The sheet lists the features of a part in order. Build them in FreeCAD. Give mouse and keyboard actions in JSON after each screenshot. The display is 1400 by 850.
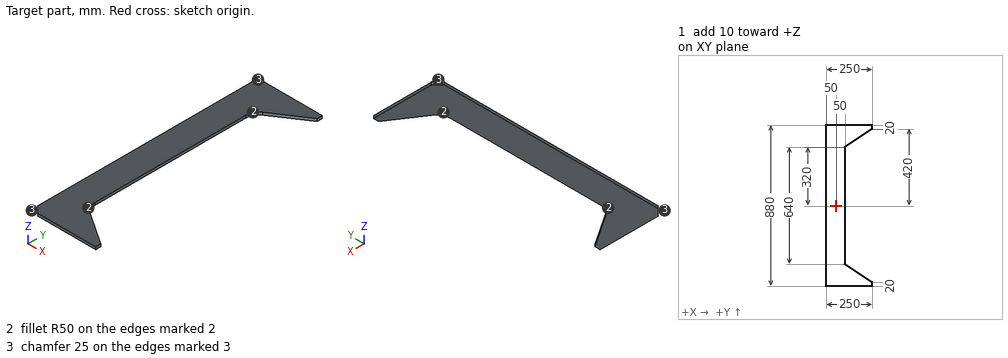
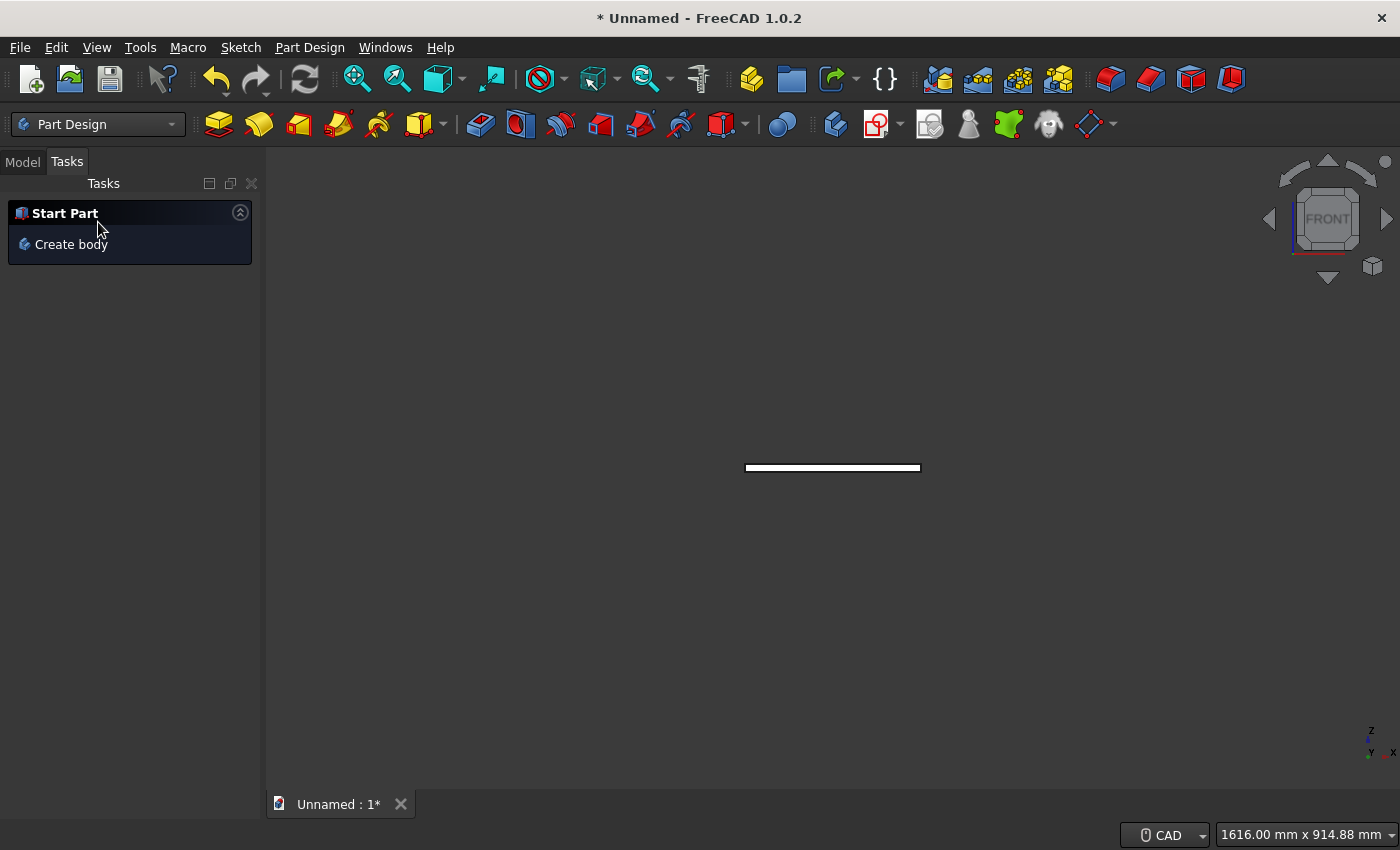
{"action": "scroll", "coordinate": [745, 467], "scroll_direction": "up", "scroll_amount": 9}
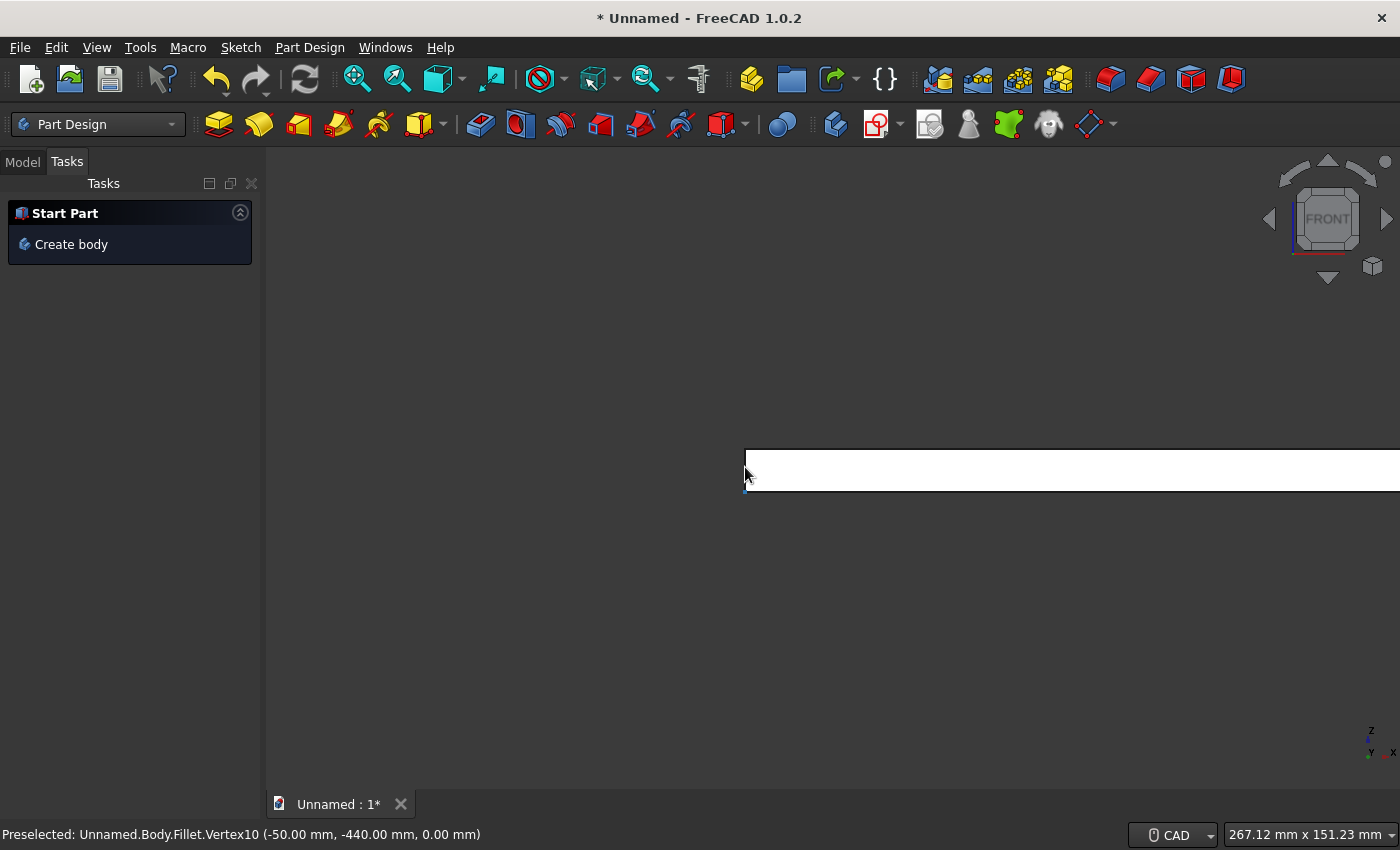
{"action": "left_click", "coordinate": [745, 470]}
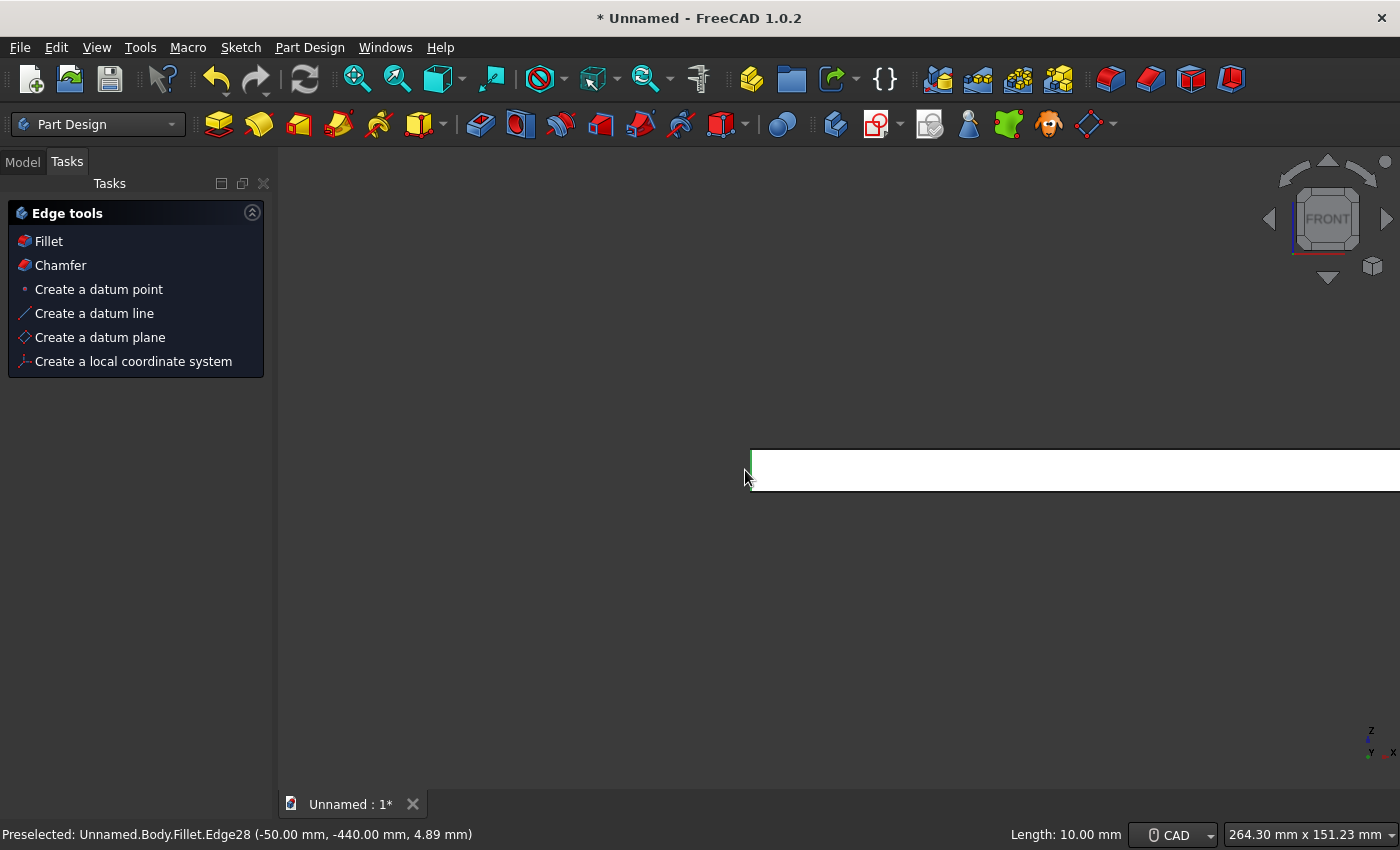
{"action": "left_click", "coordinate": [358, 80]}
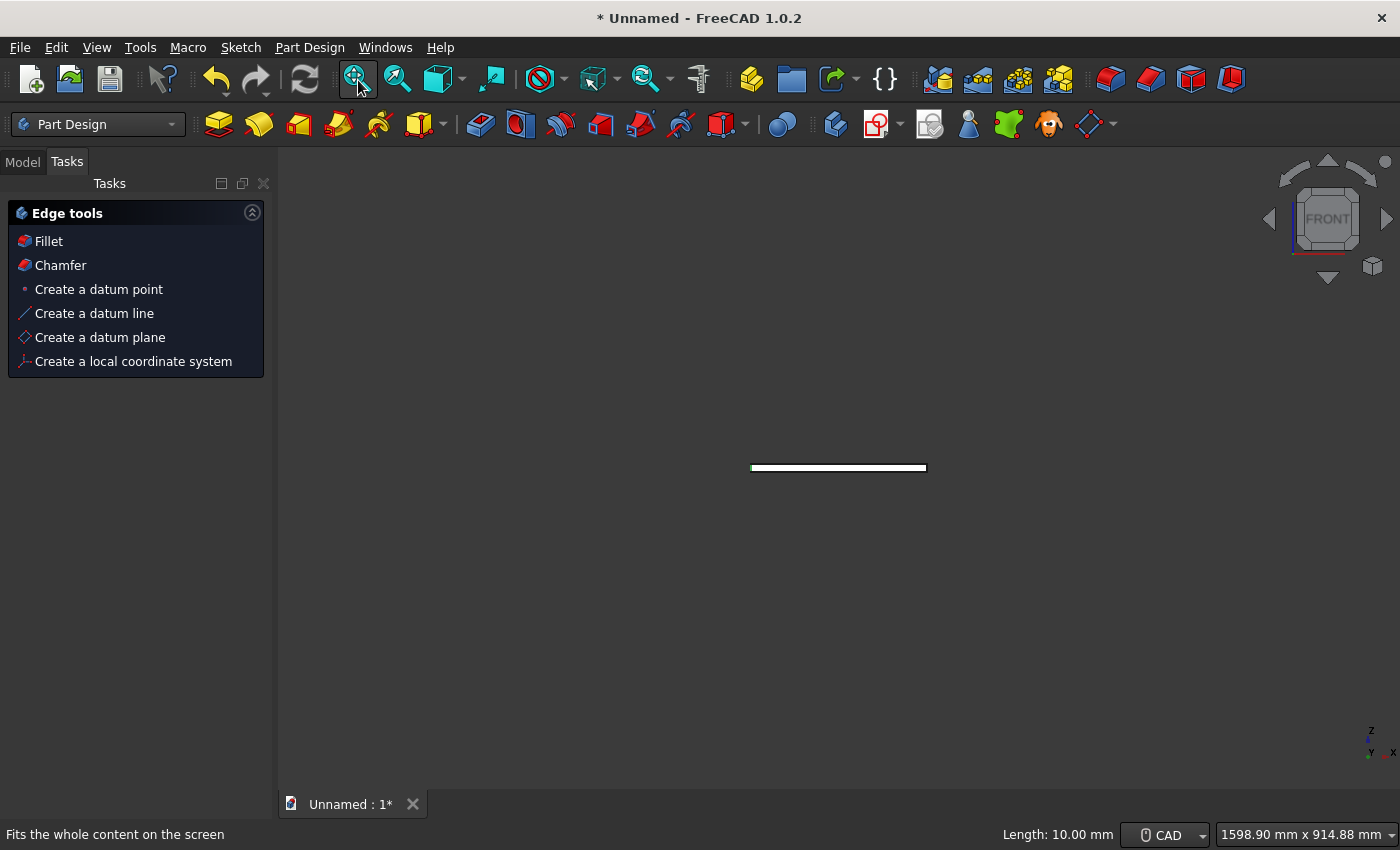
{"action": "key", "text": "0"}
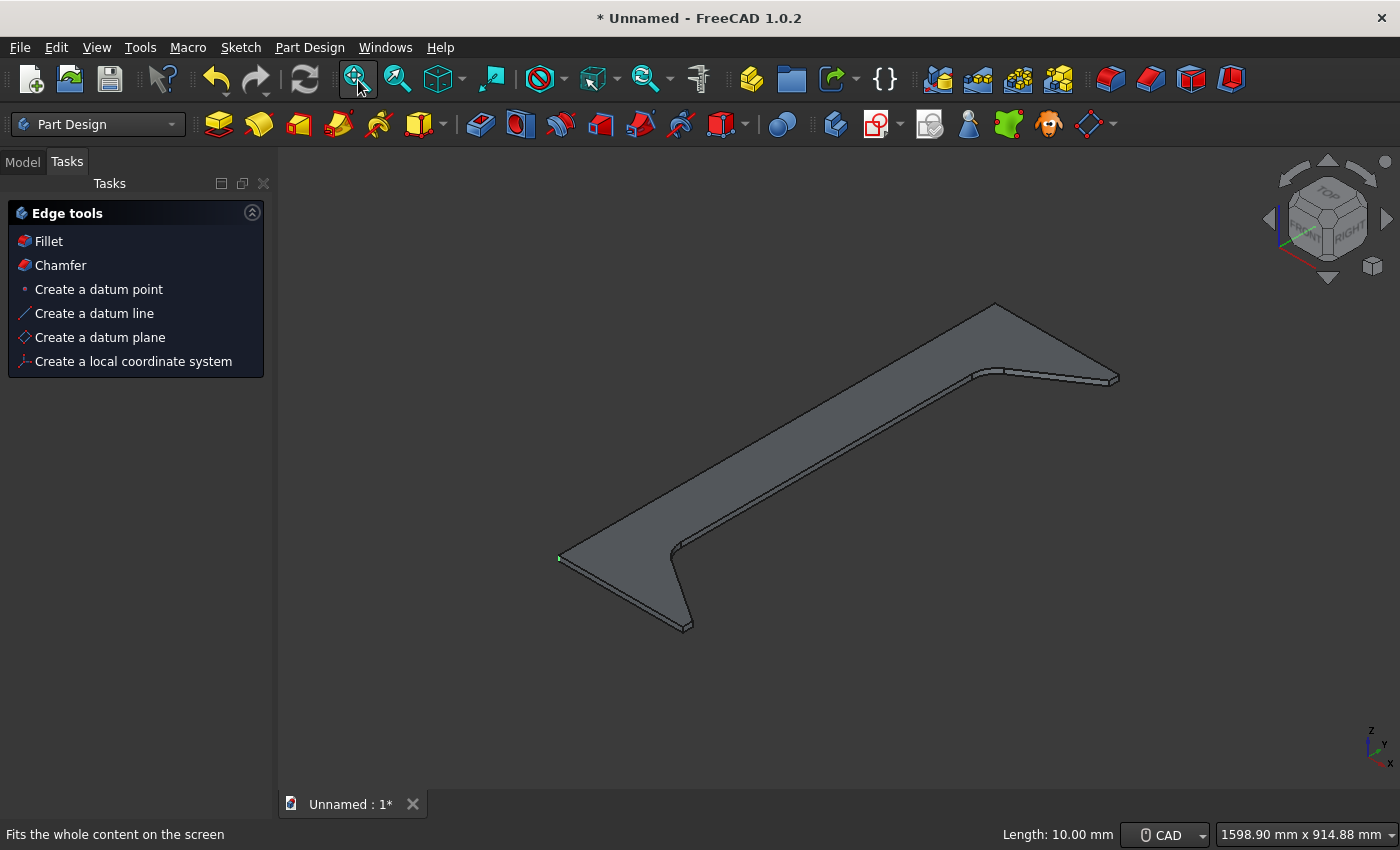
{"action": "scroll", "coordinate": [995, 305], "scroll_direction": "up", "scroll_amount": 9}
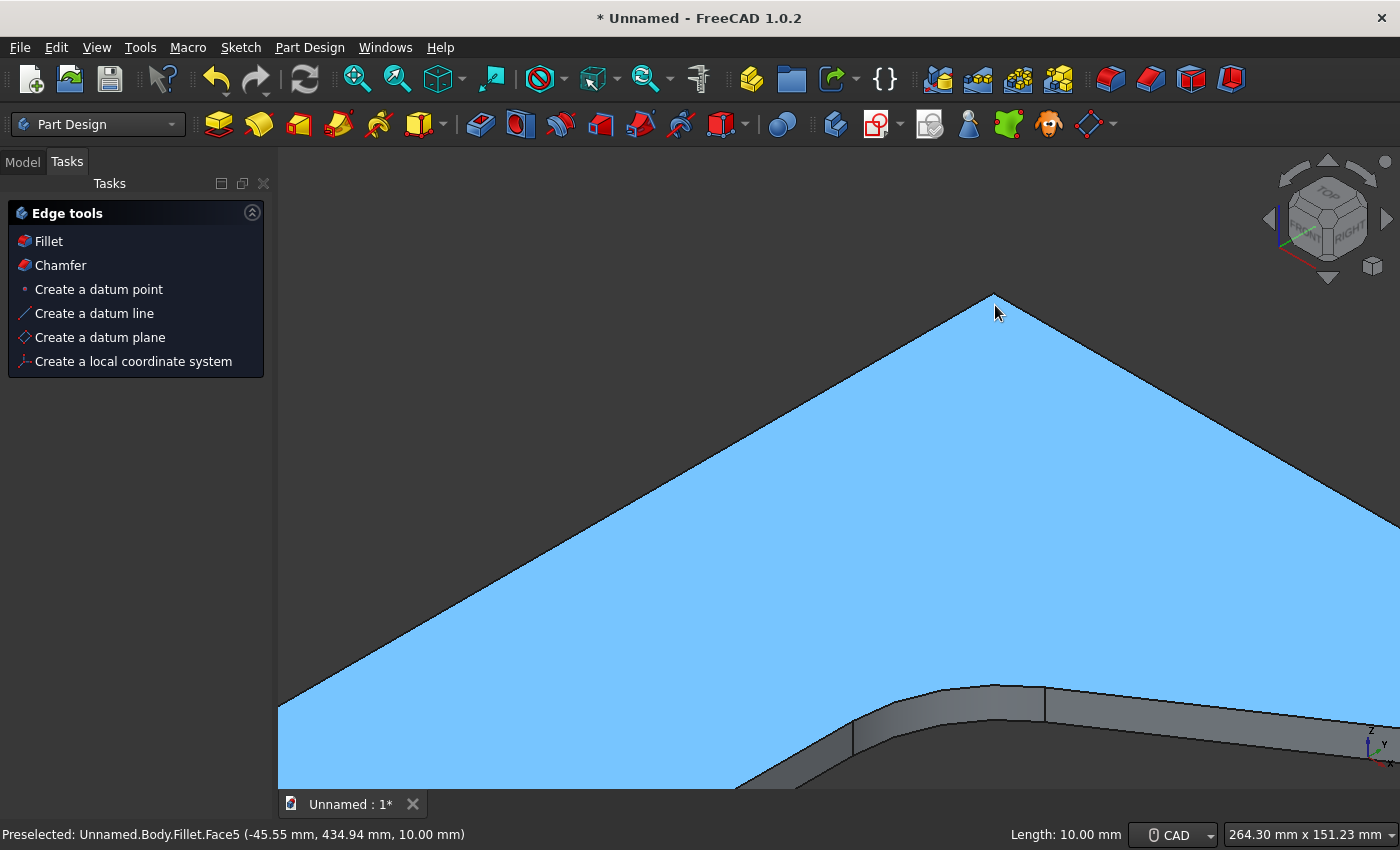
{"action": "key", "text": "v f"}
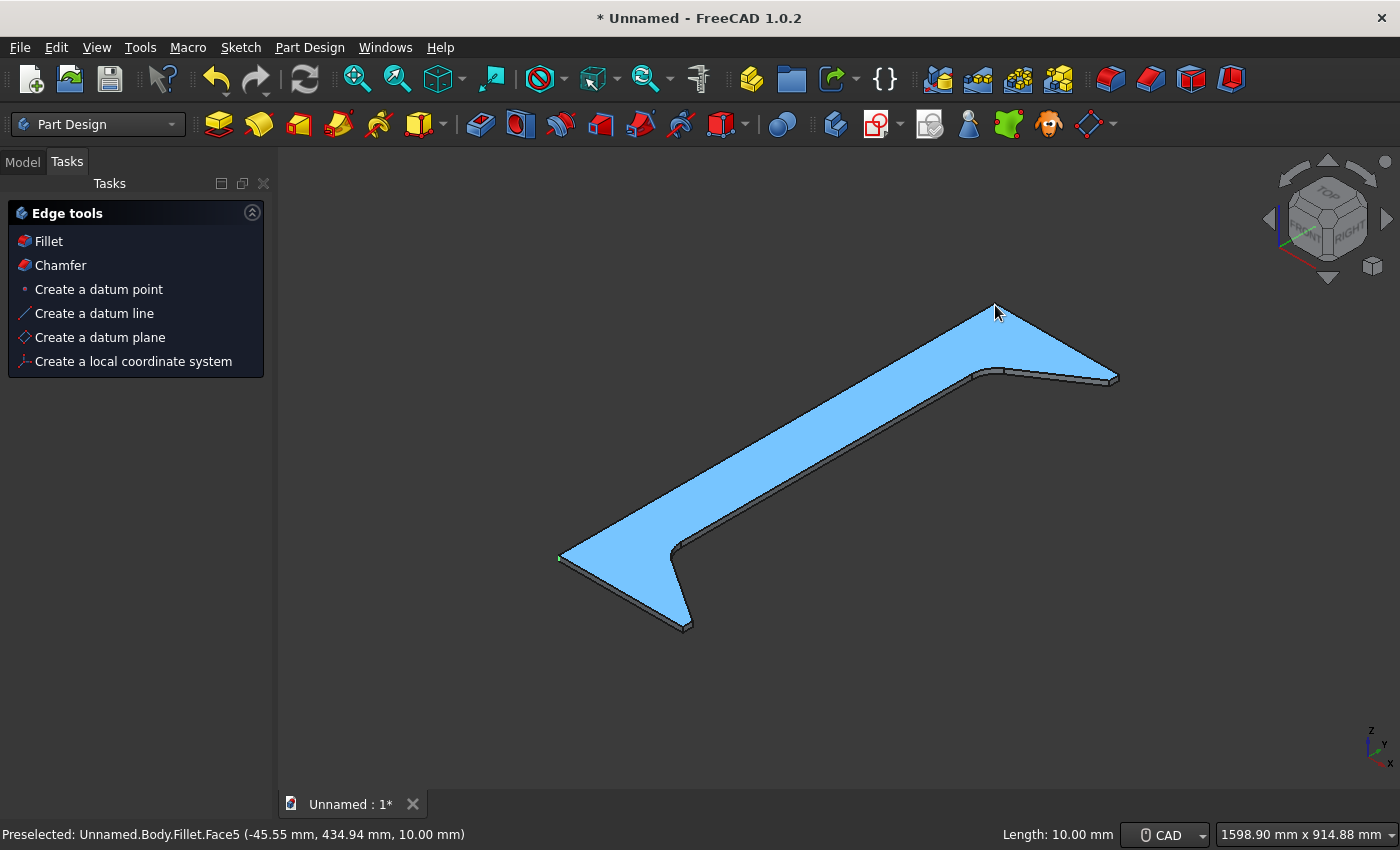
{"action": "key", "text": "2"}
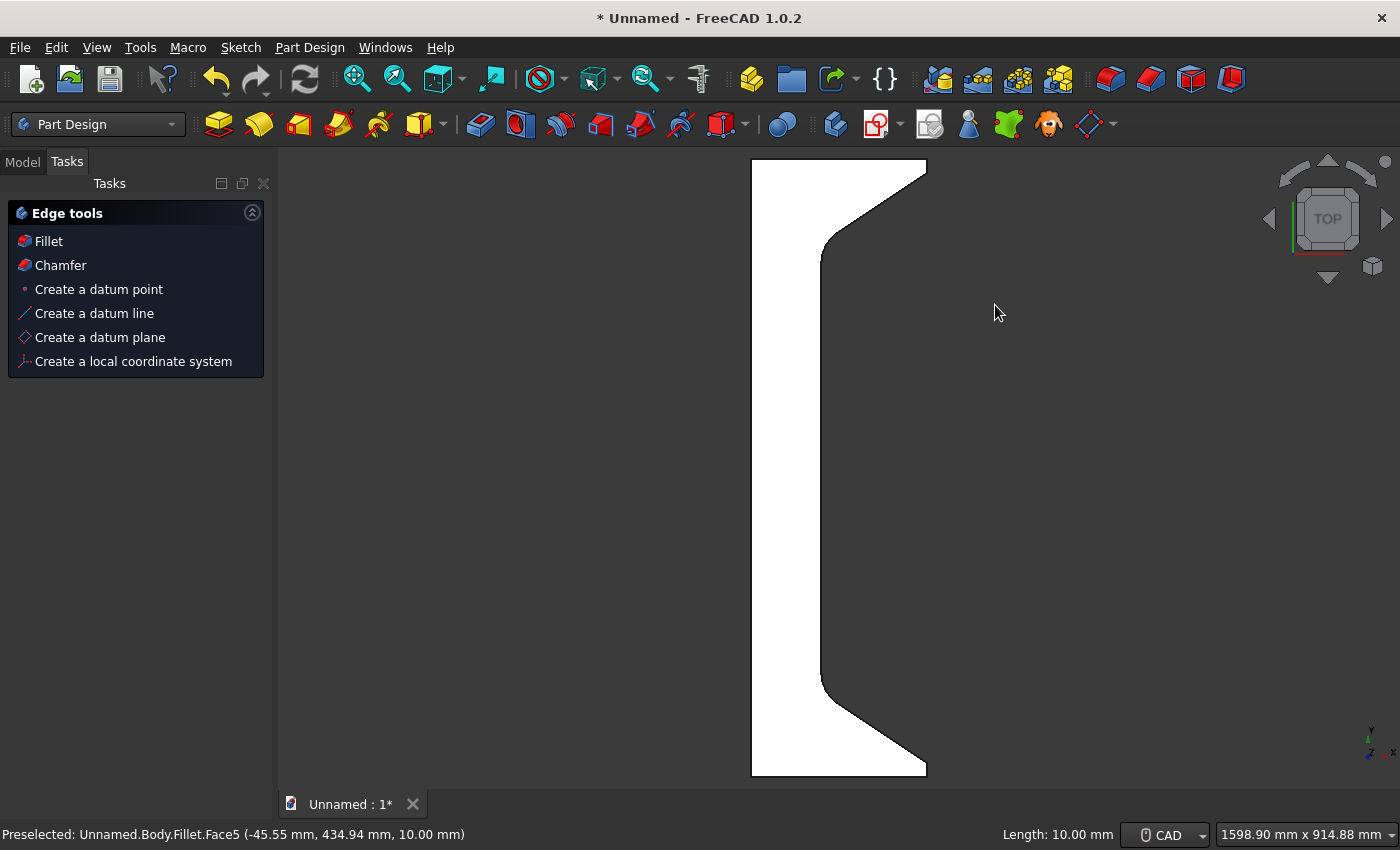
{"action": "key", "text": "1"}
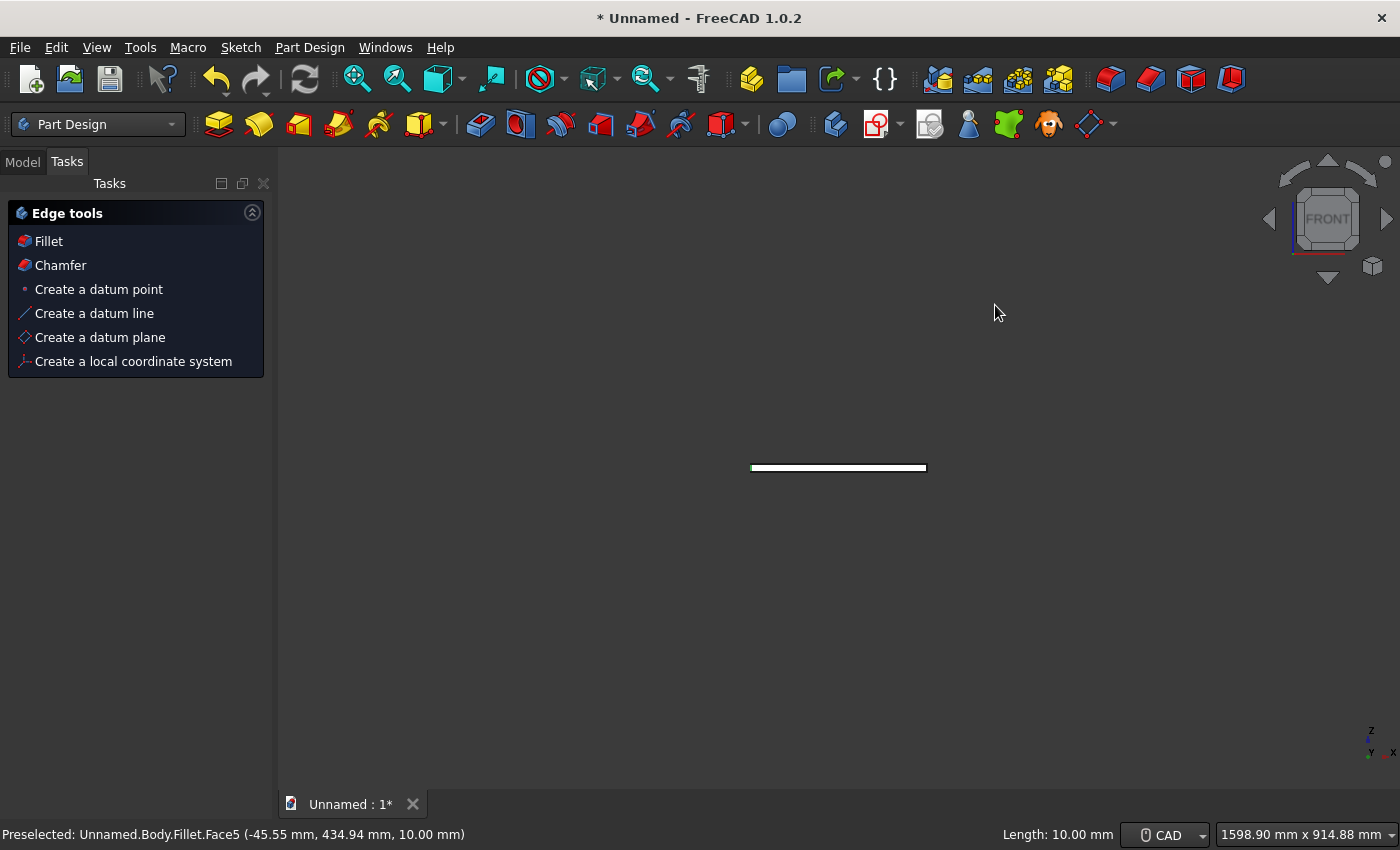
{"action": "left_click", "coordinate": [358, 80]}